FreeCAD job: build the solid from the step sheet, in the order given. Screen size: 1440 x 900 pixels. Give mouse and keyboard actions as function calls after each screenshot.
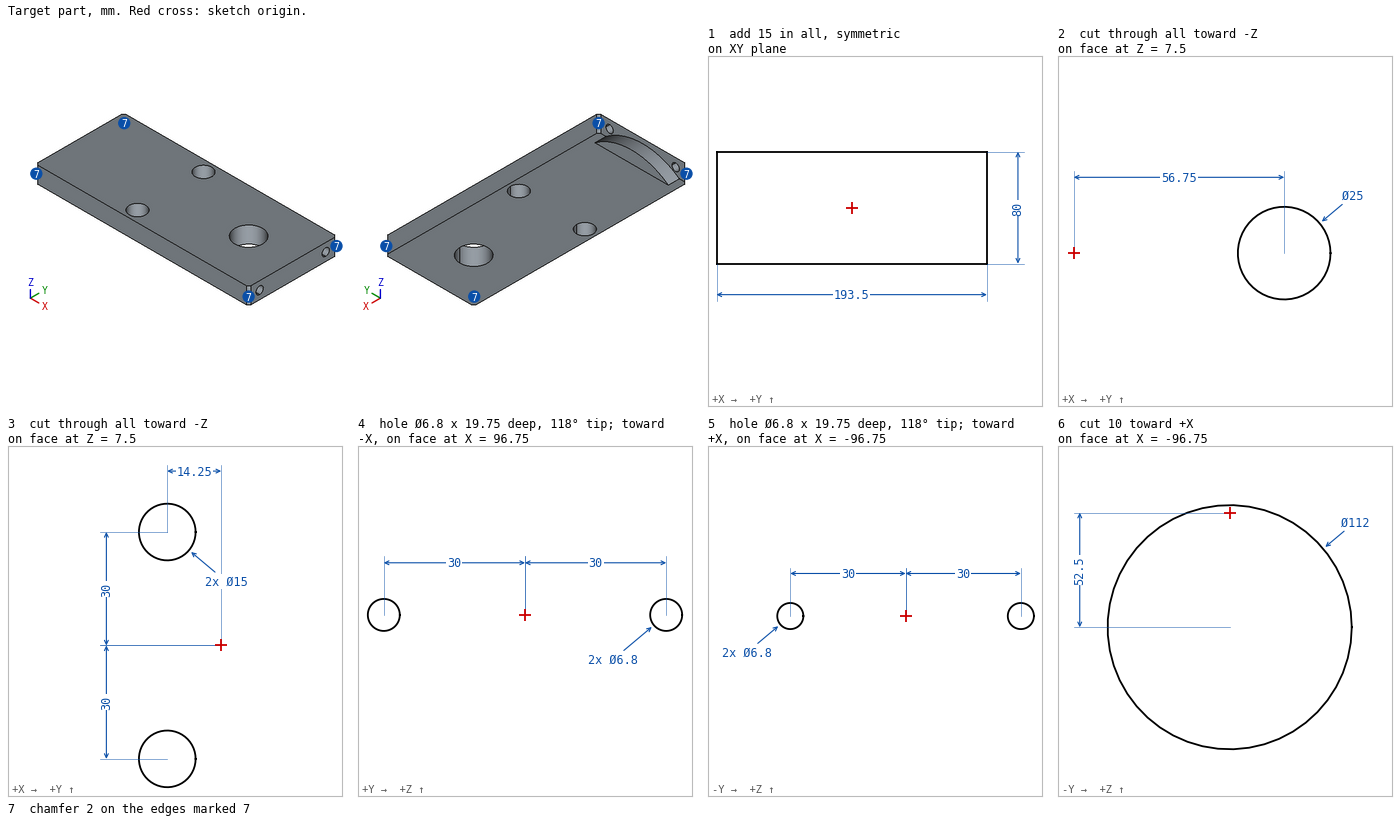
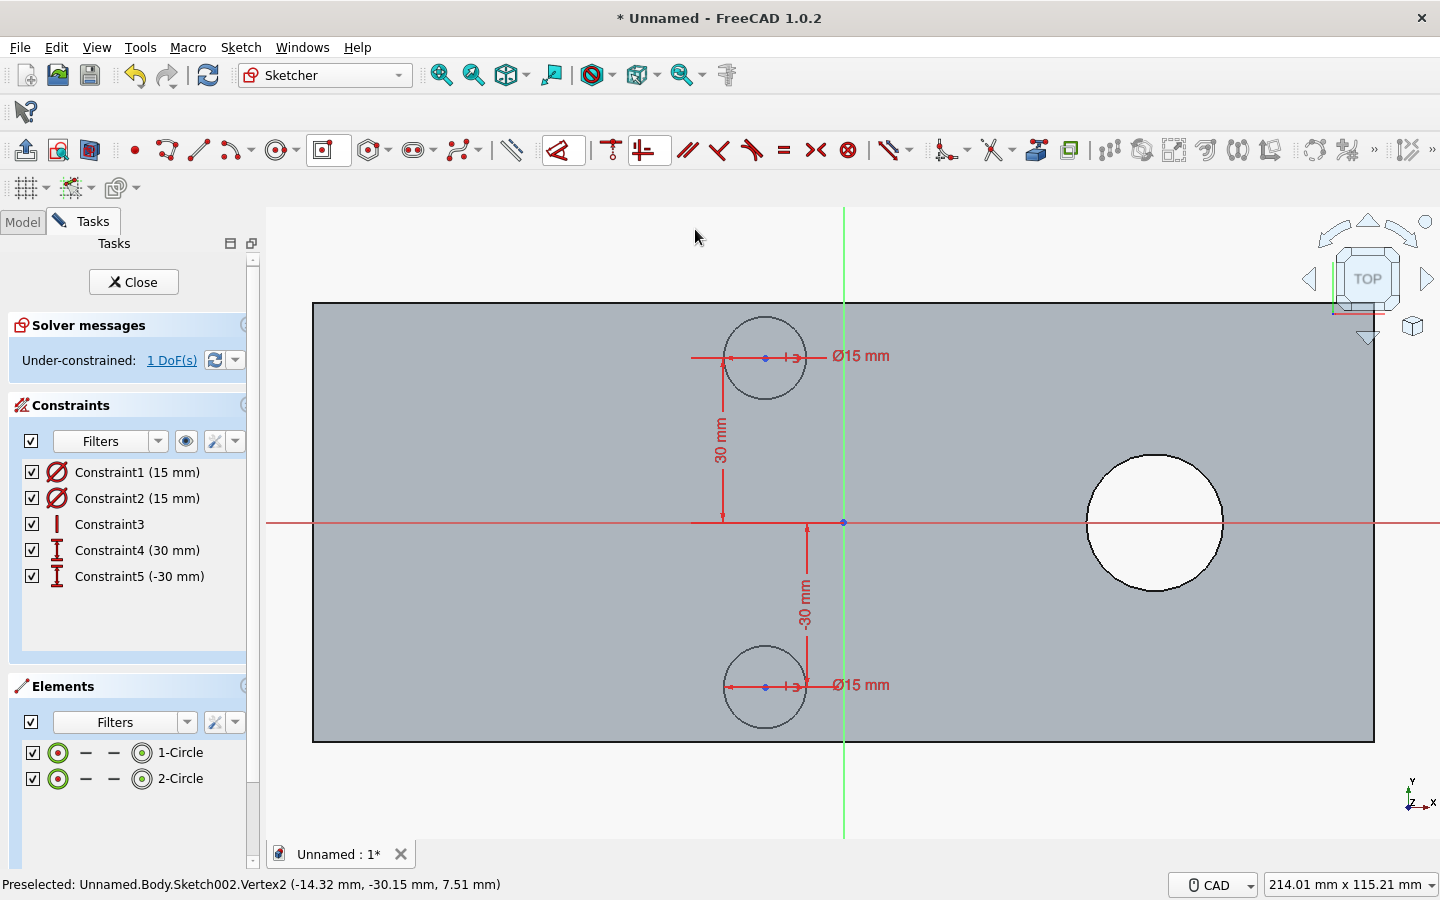
click(765, 358)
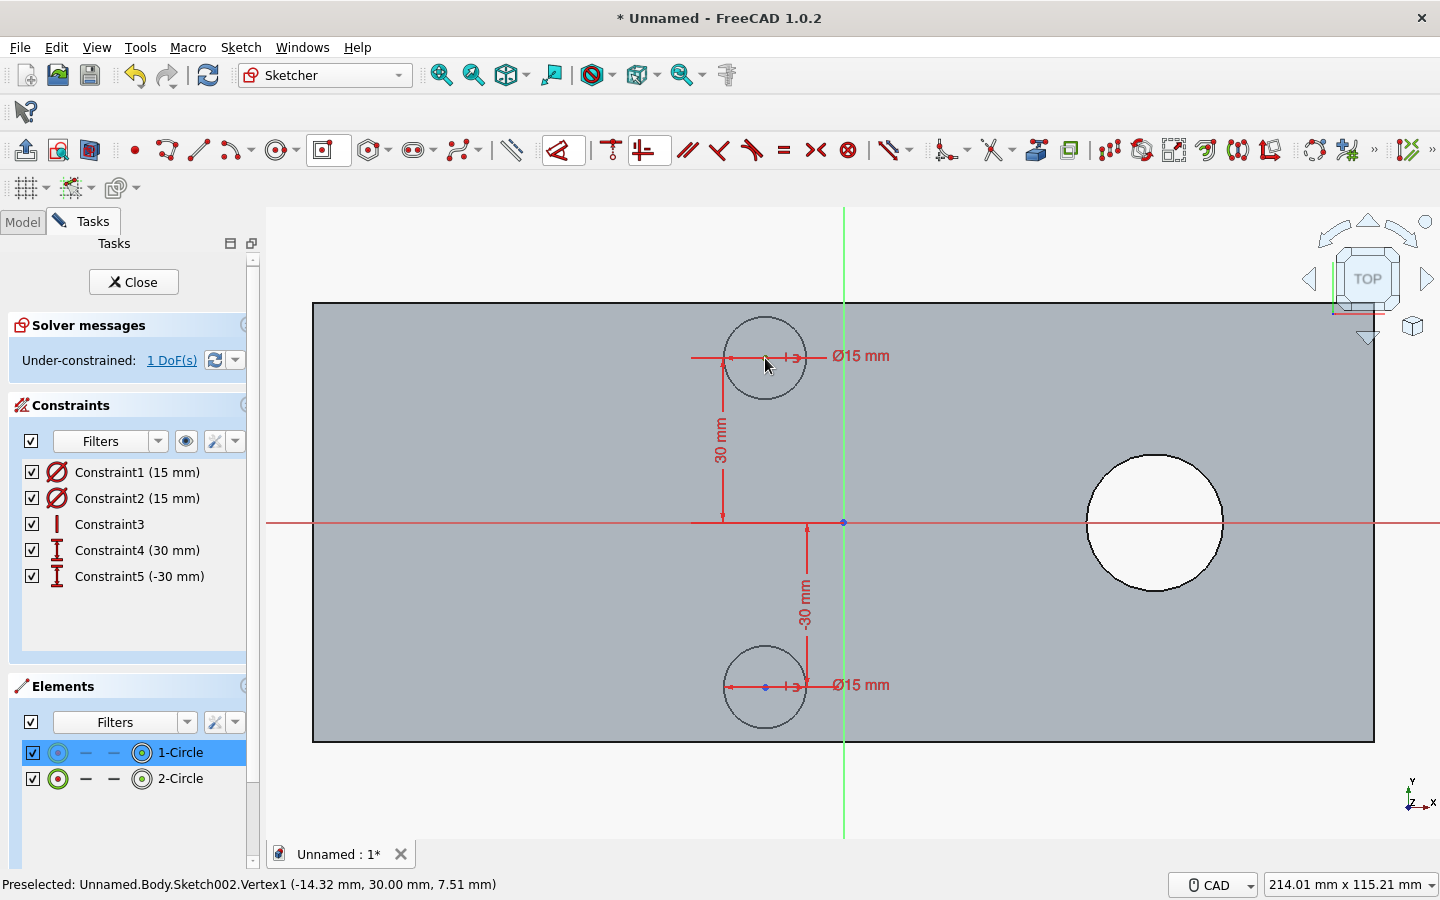
click(580, 150)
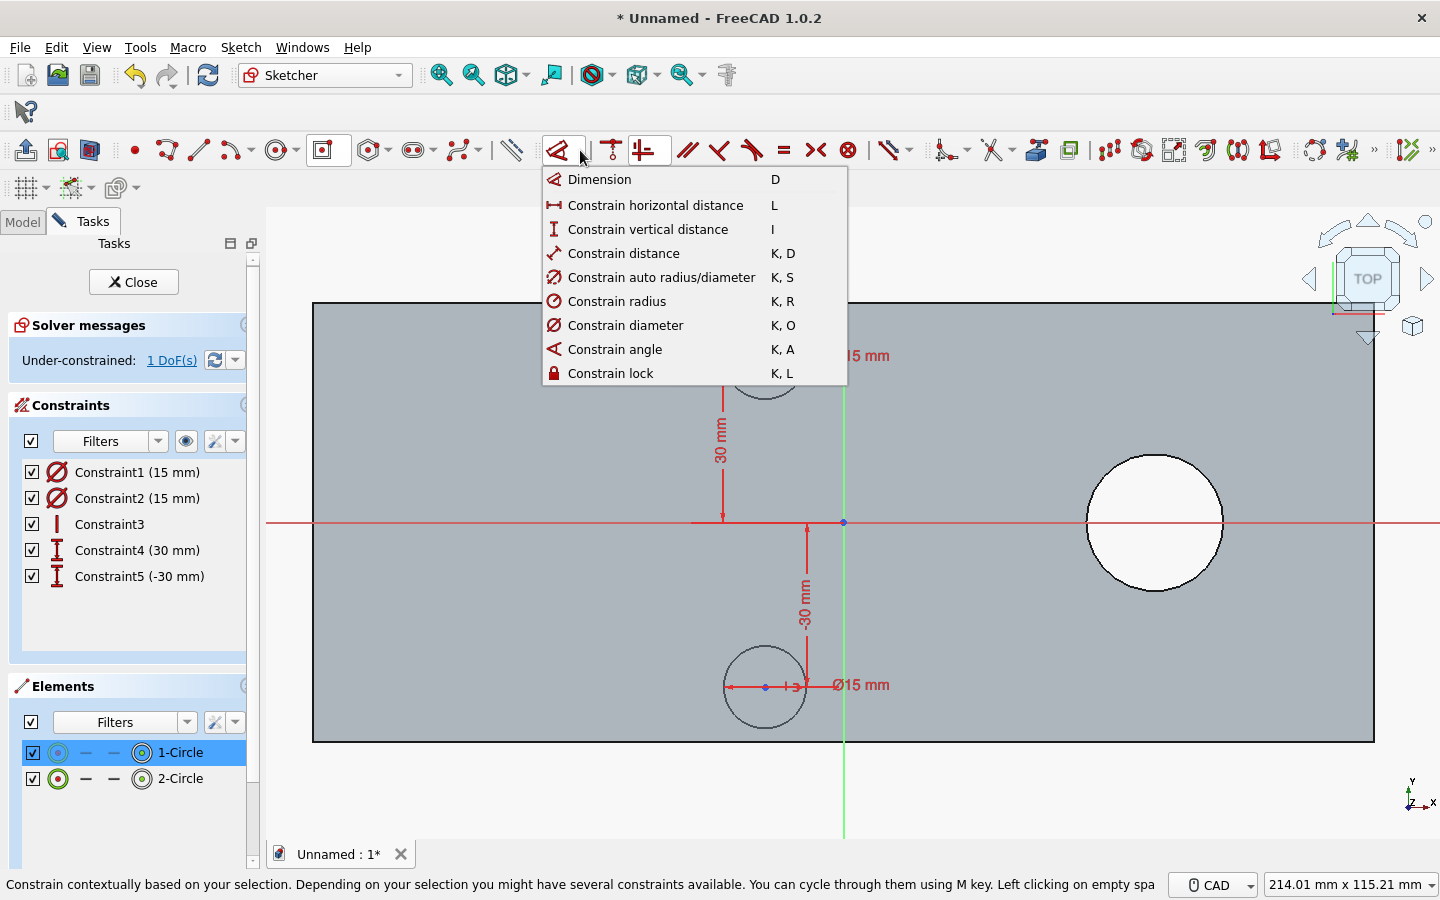
click(695, 205)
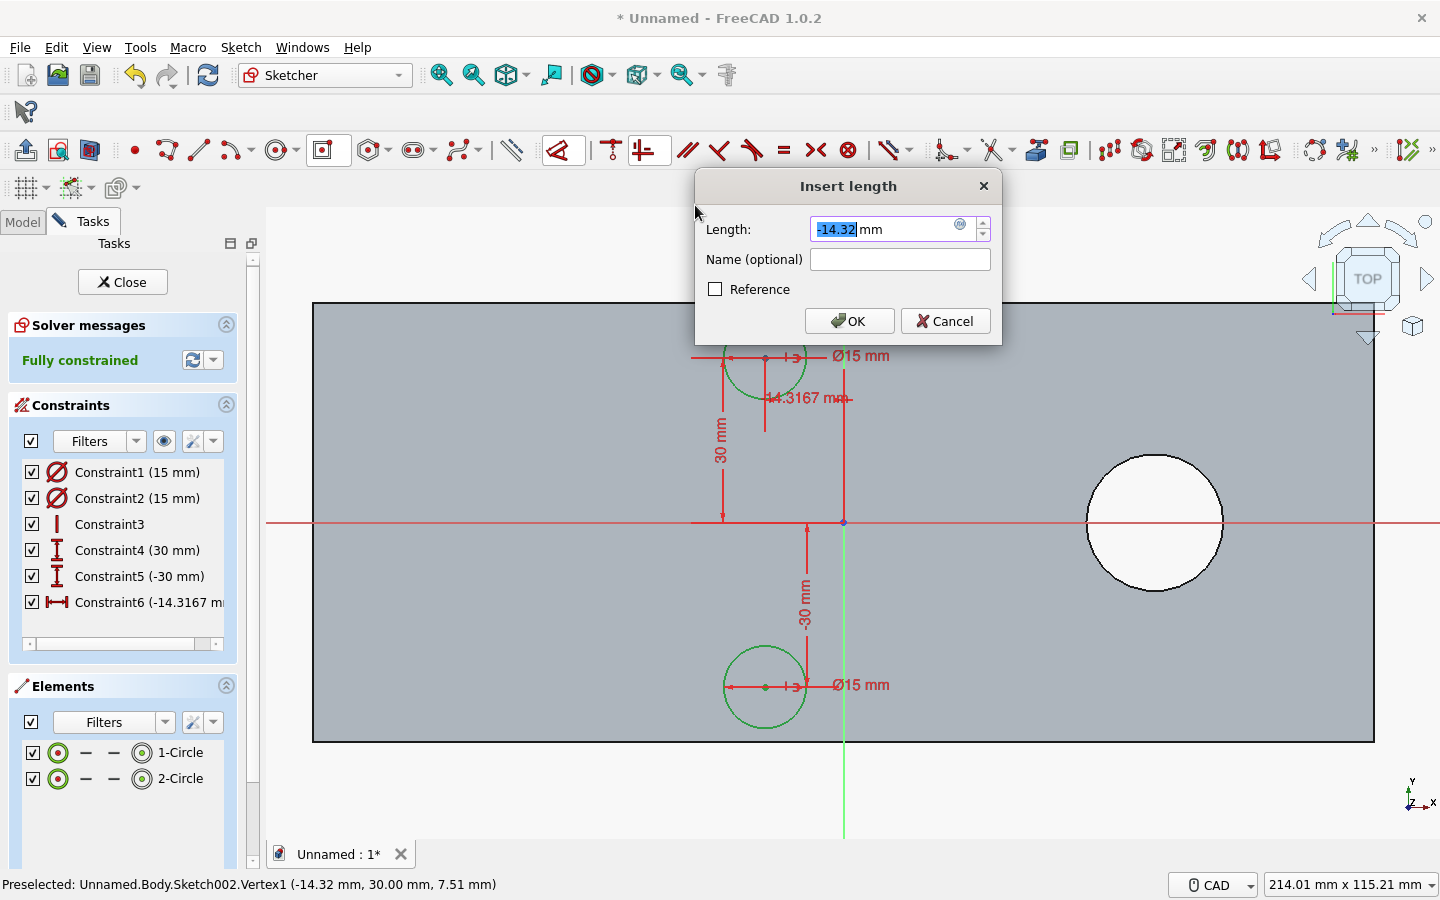
text(-14.25)
key(Return)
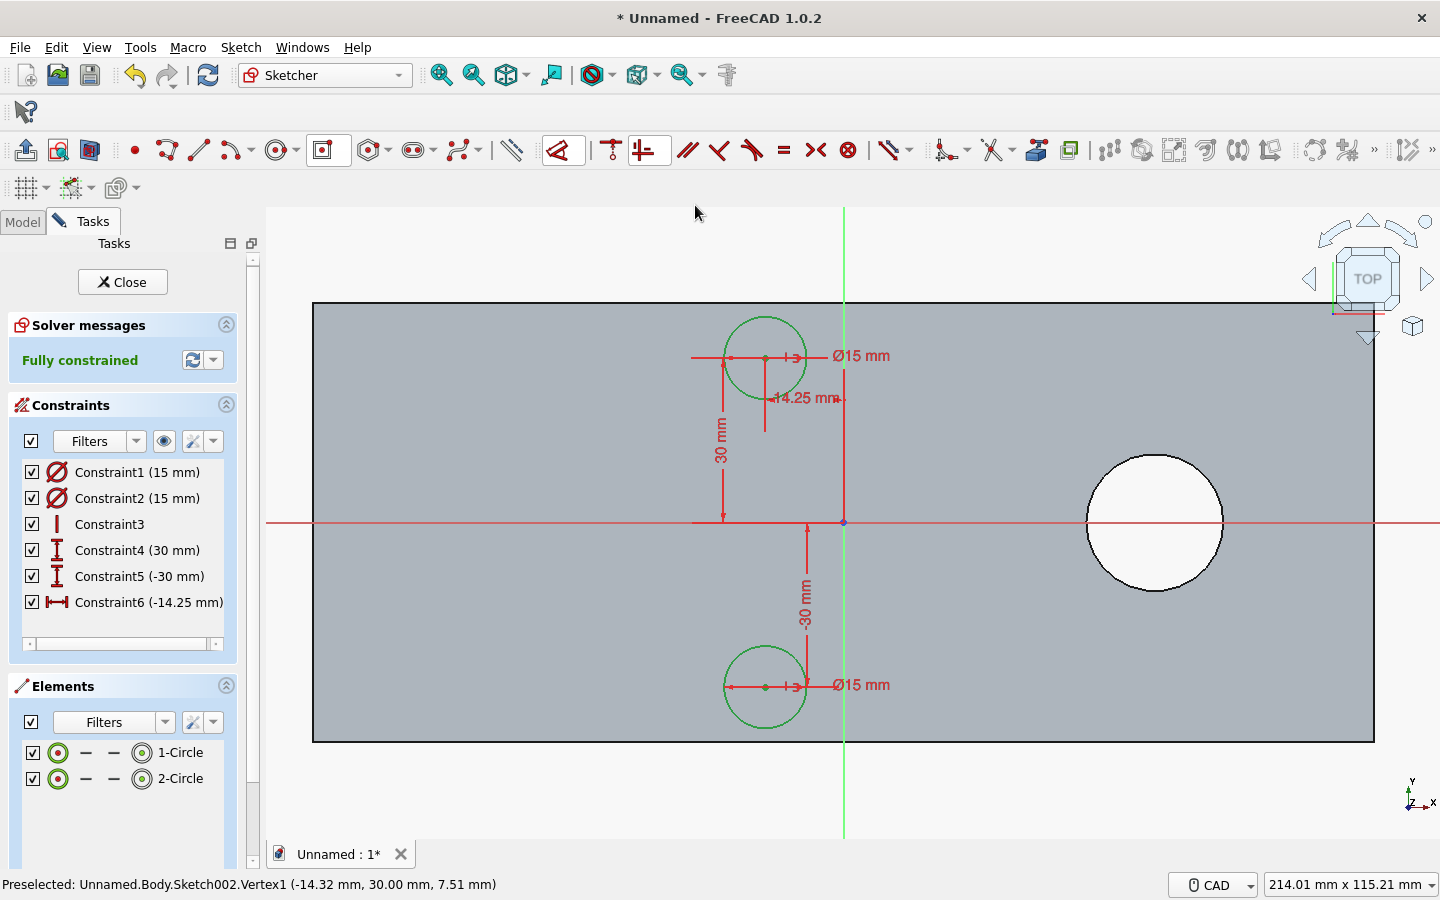
click(123, 282)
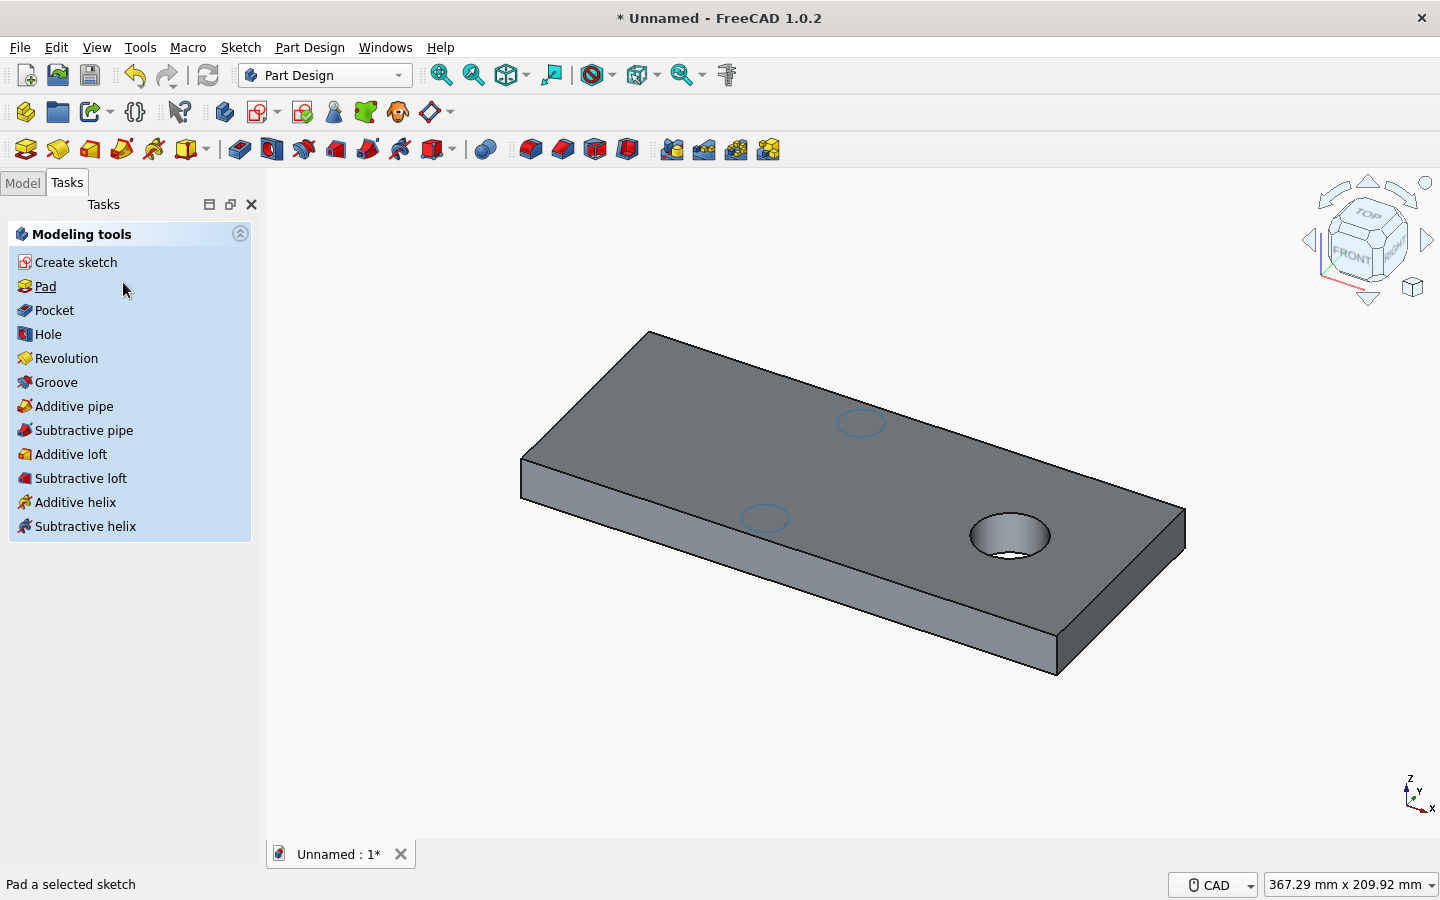
click(240, 150)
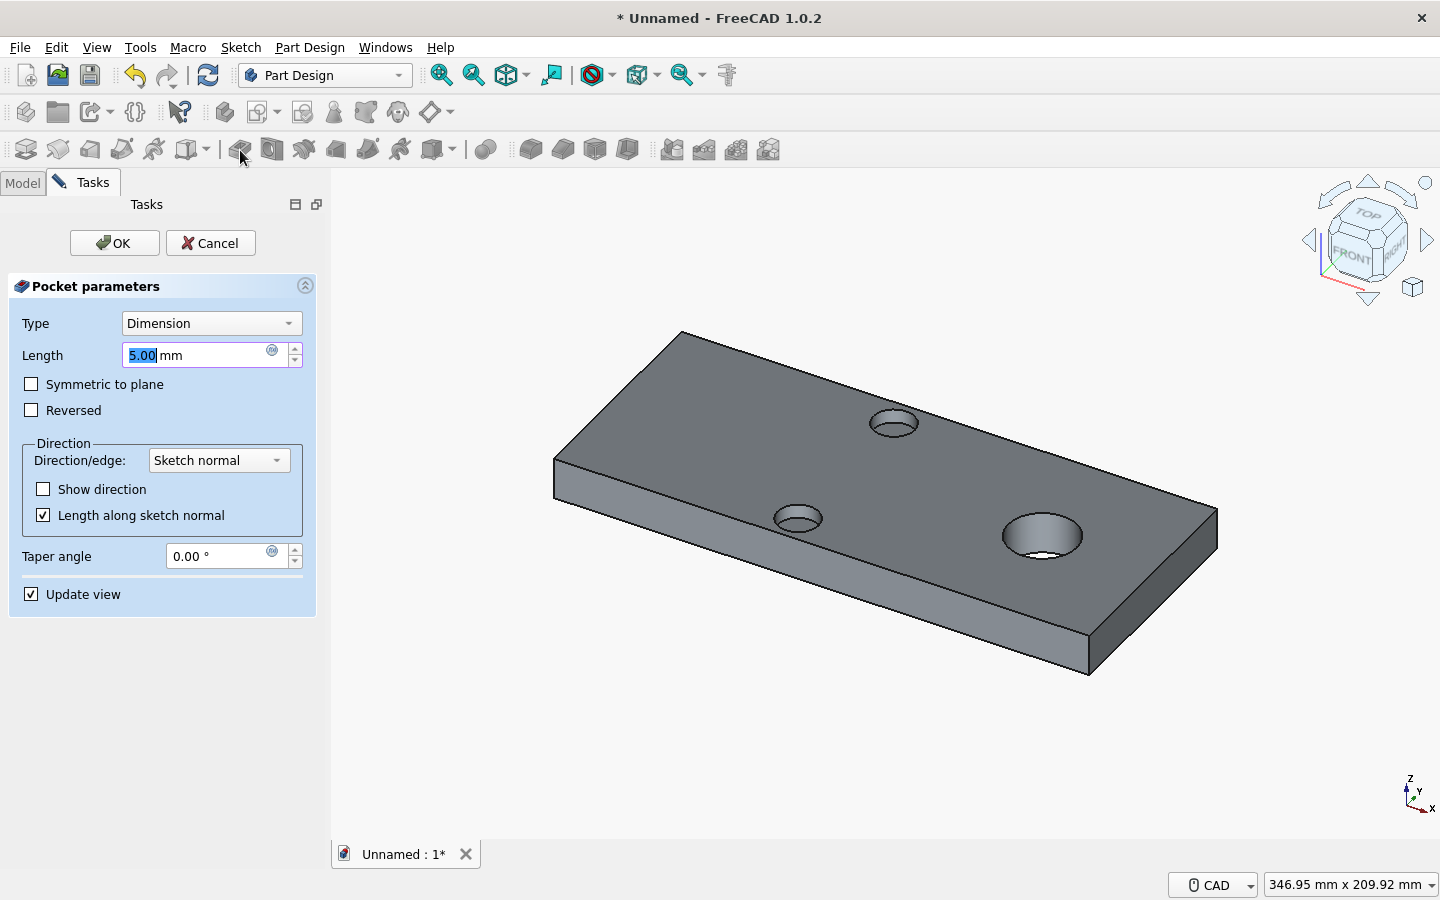
click(212, 324)